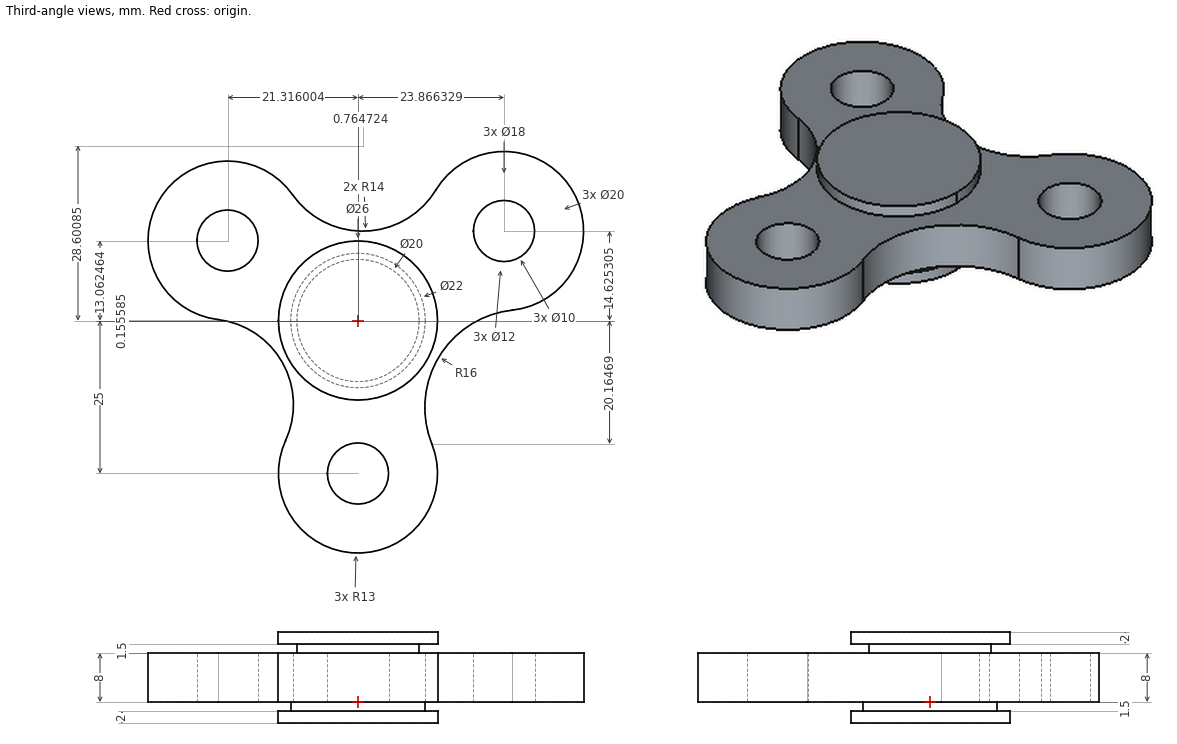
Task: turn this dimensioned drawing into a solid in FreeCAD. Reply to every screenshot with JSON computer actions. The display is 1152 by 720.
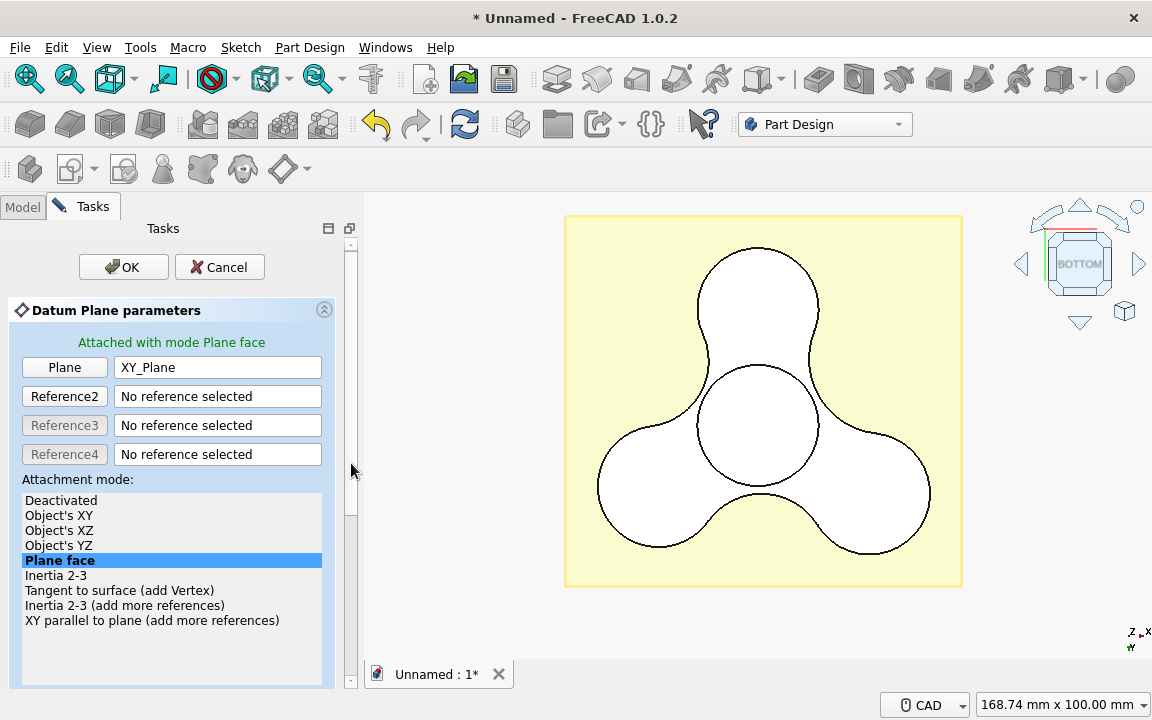
{"action": "left_click", "coordinate": [124, 267]}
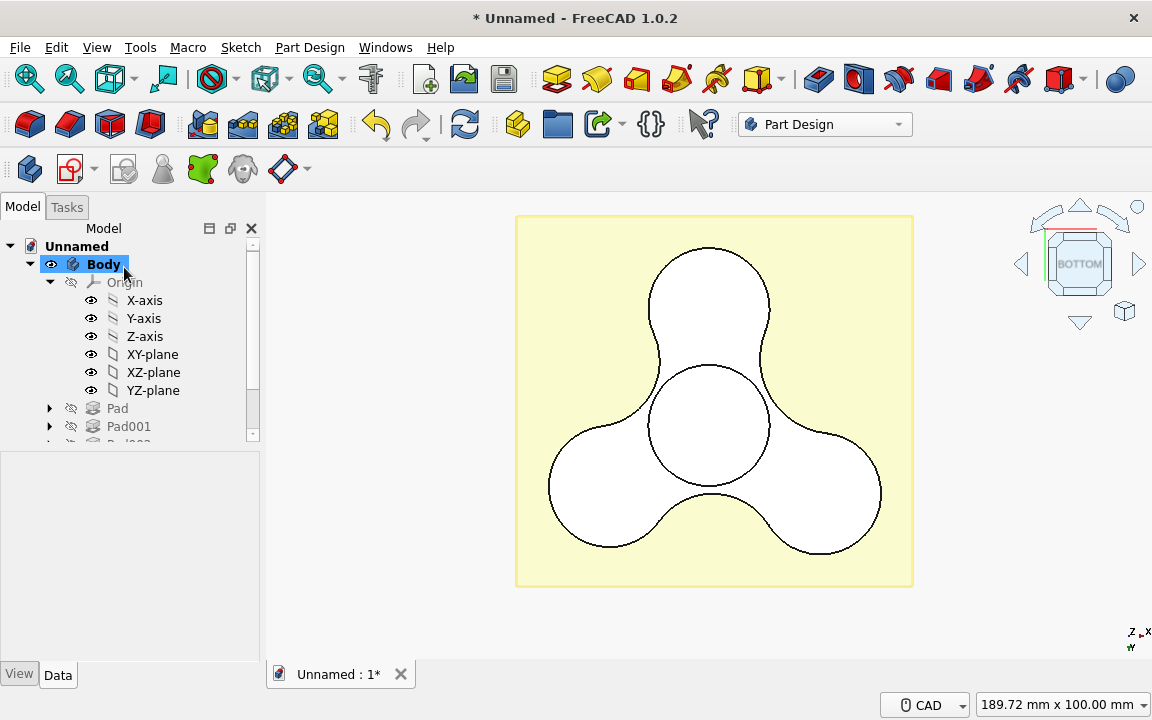
{"action": "scroll", "coordinate": [100, 332], "scroll_direction": "down", "scroll_amount": 3}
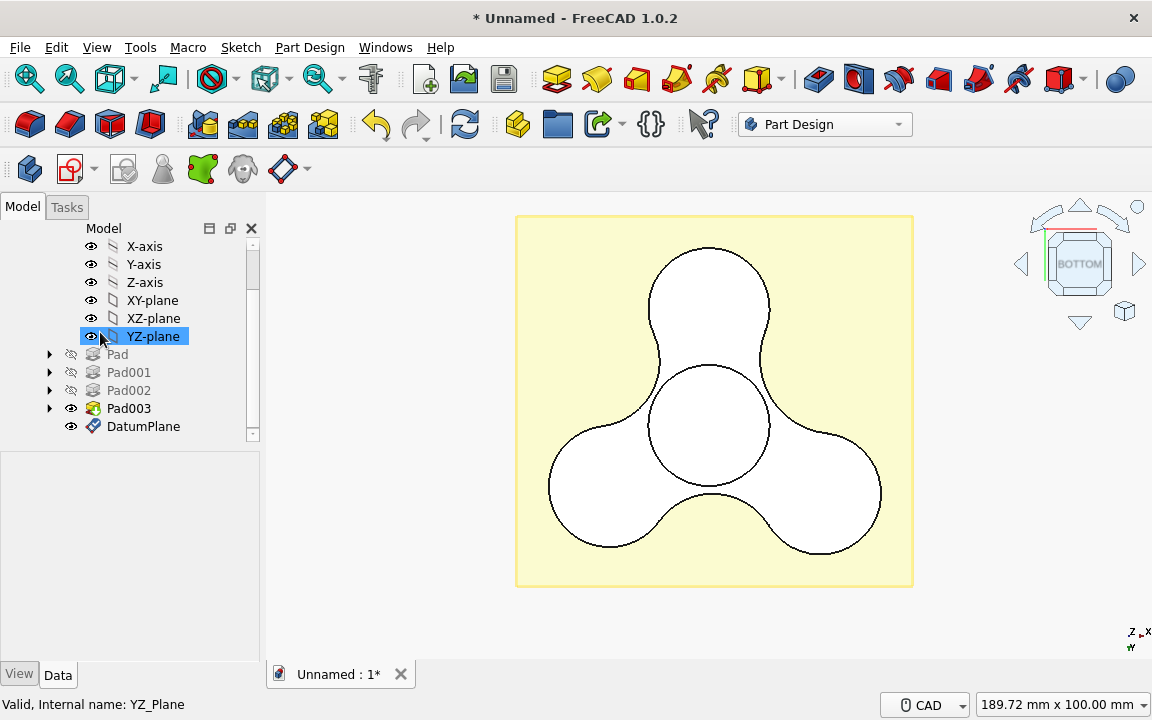
{"action": "left_click", "coordinate": [116, 426]}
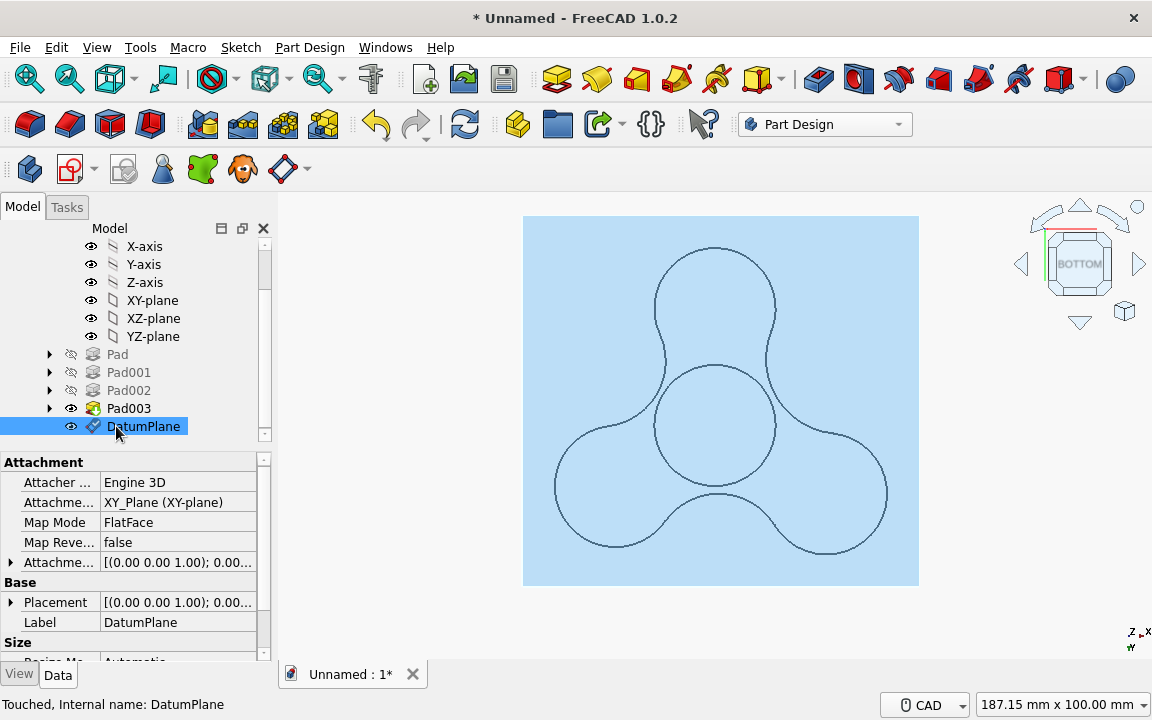
{"action": "left_click", "coordinate": [70, 170]}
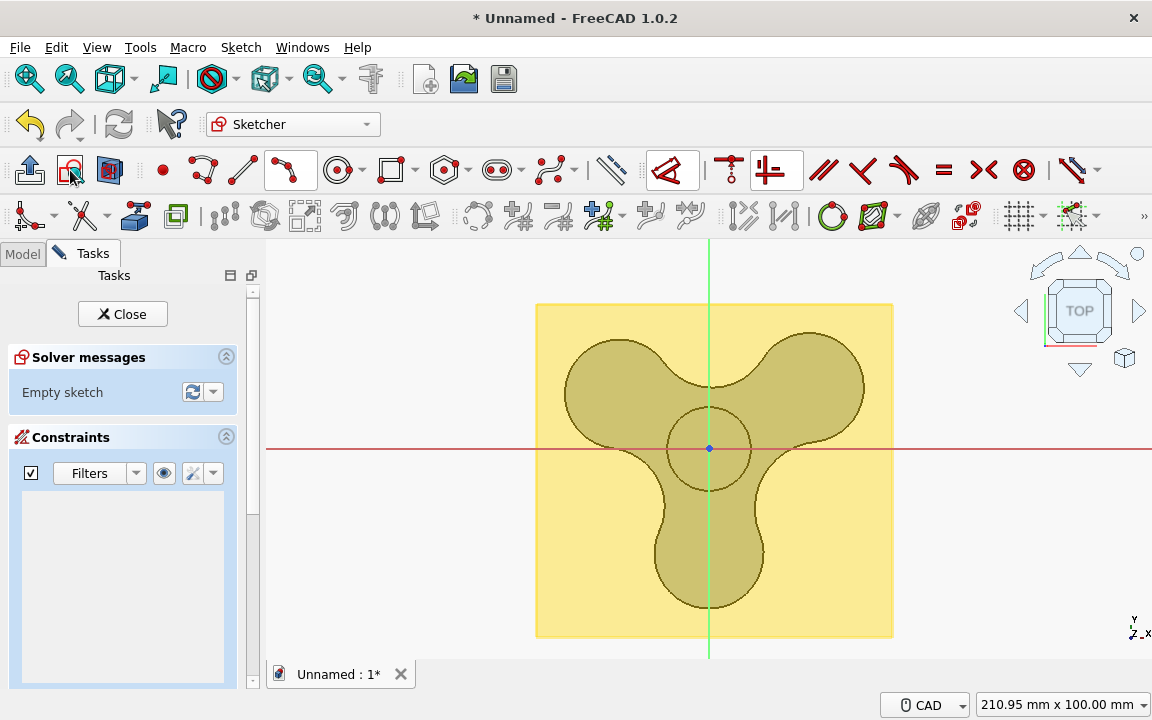
{"action": "scroll", "coordinate": [765, 449], "scroll_direction": "up", "scroll_amount": 4}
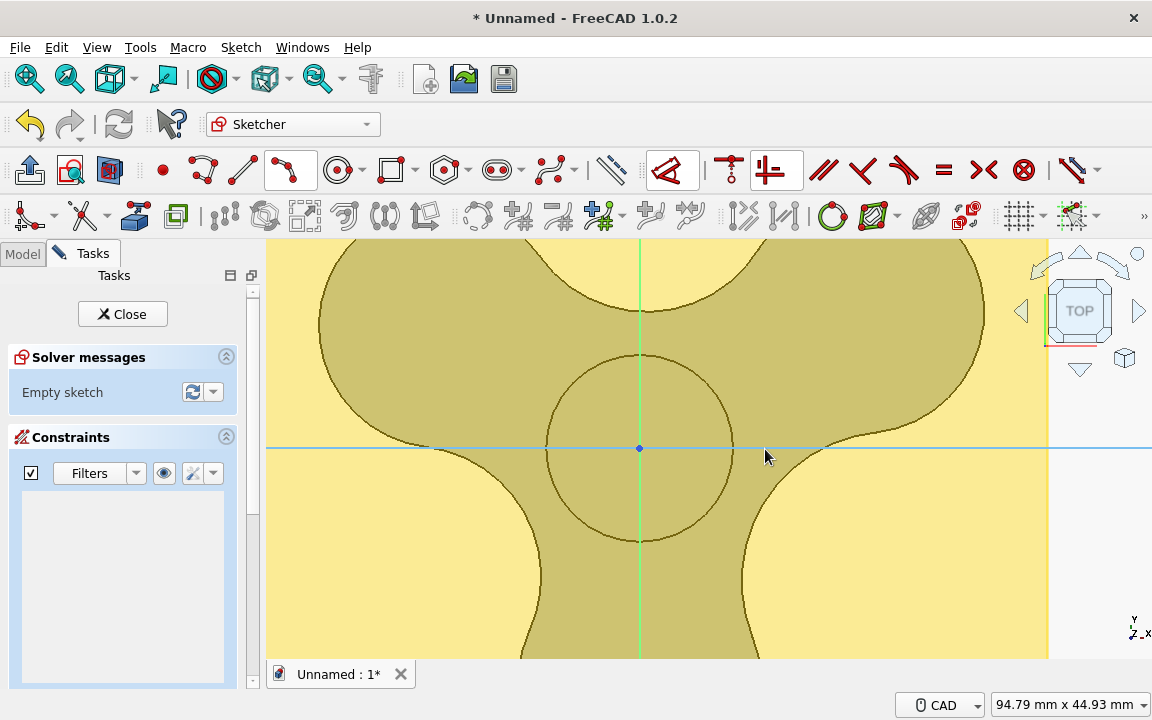
{"action": "left_click", "coordinate": [338, 170]}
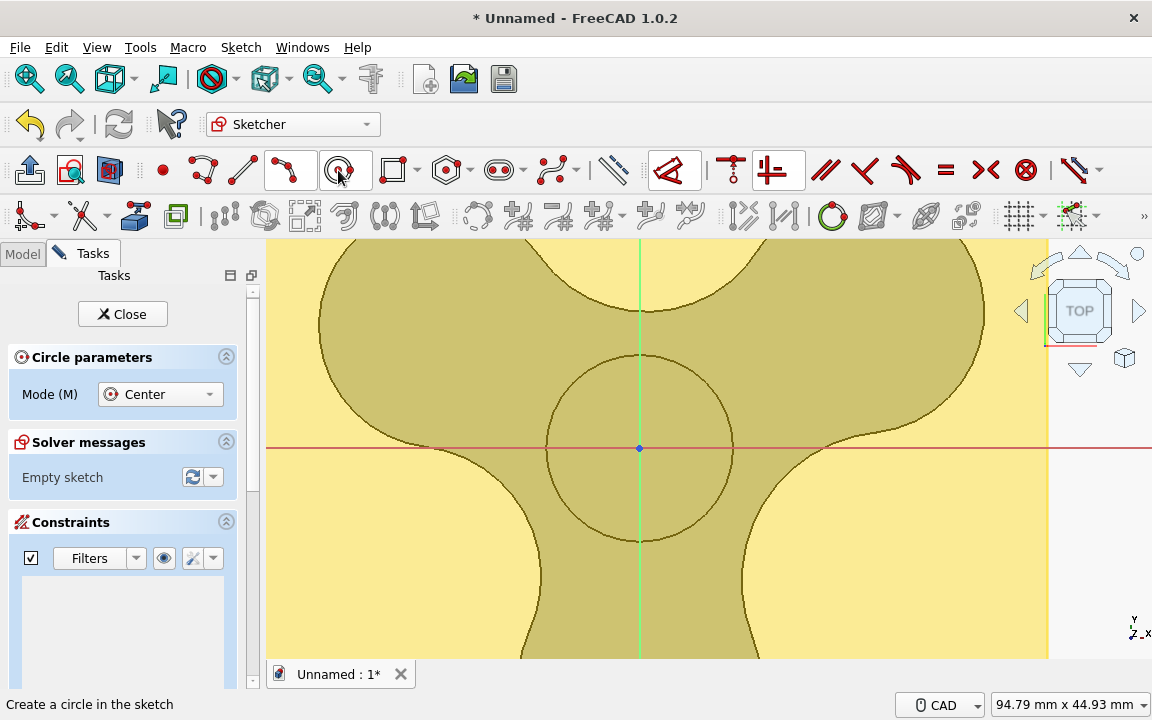
{"action": "left_click", "coordinate": [640, 448]}
{"action": "mouse_move", "coordinate": [726, 362]}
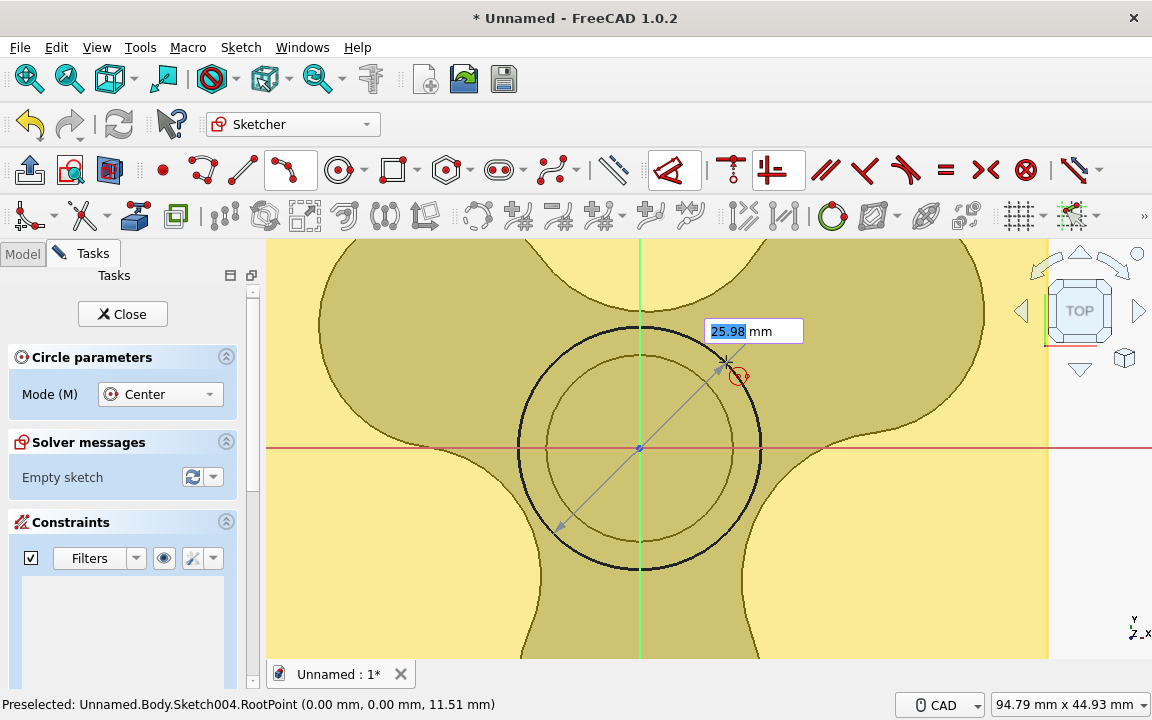
{"action": "type", "text": "26"}
{"action": "key", "text": "Return"}
{"action": "key", "text": "Escape"}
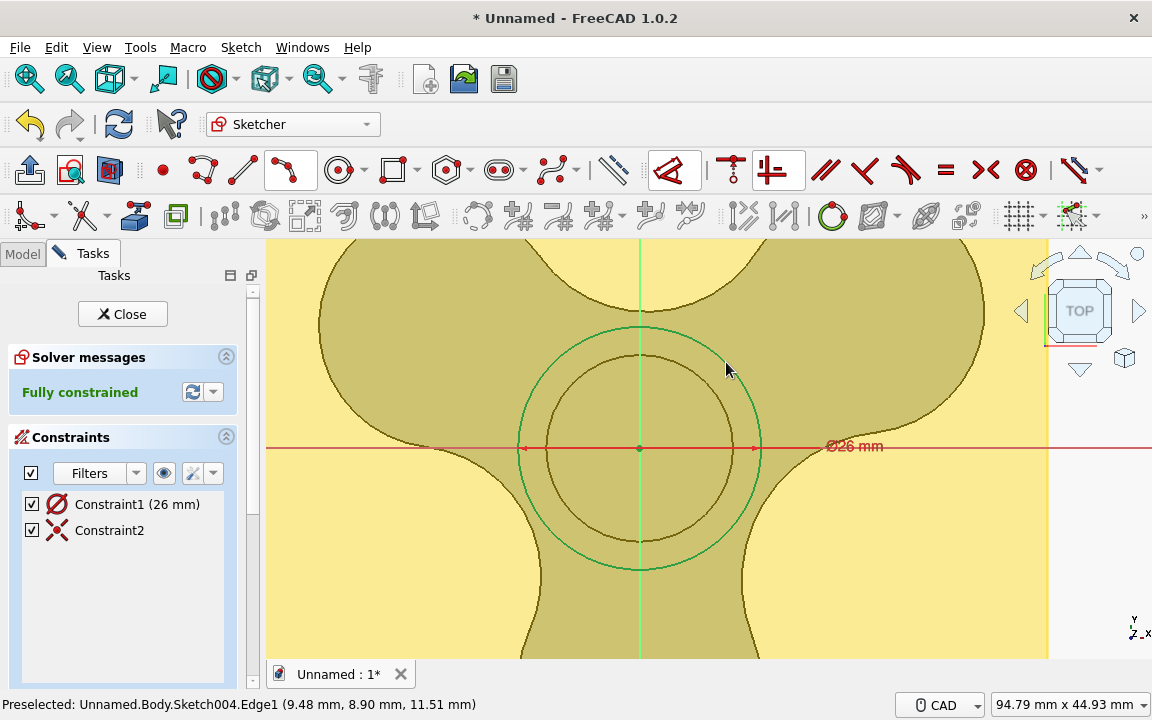
{"action": "left_click", "coordinate": [123, 314]}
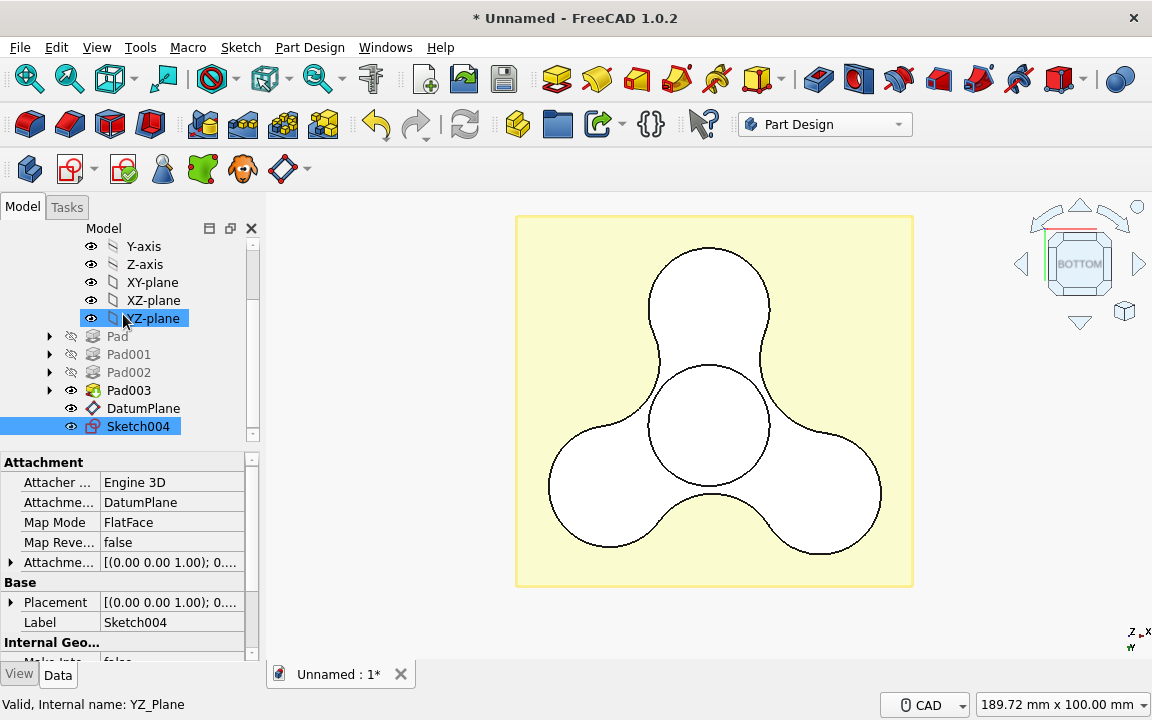
{"action": "left_click", "coordinate": [558, 80]}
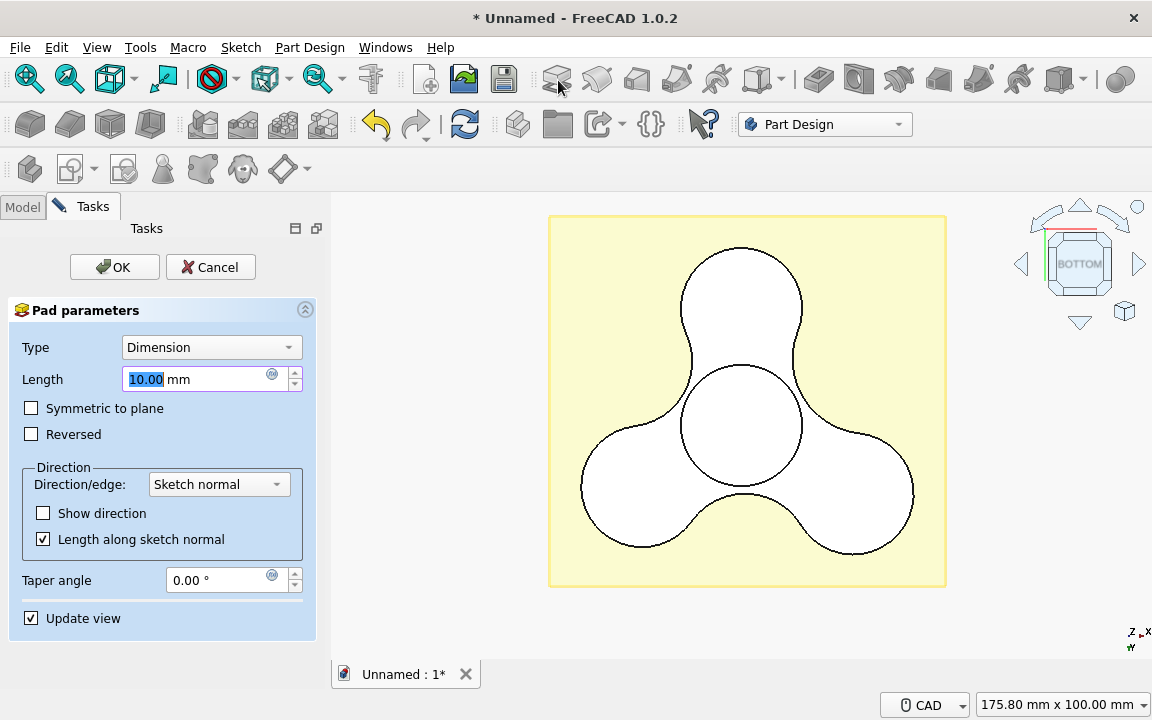
{"action": "type", "text": "2"}
{"action": "key", "text": "Tab"}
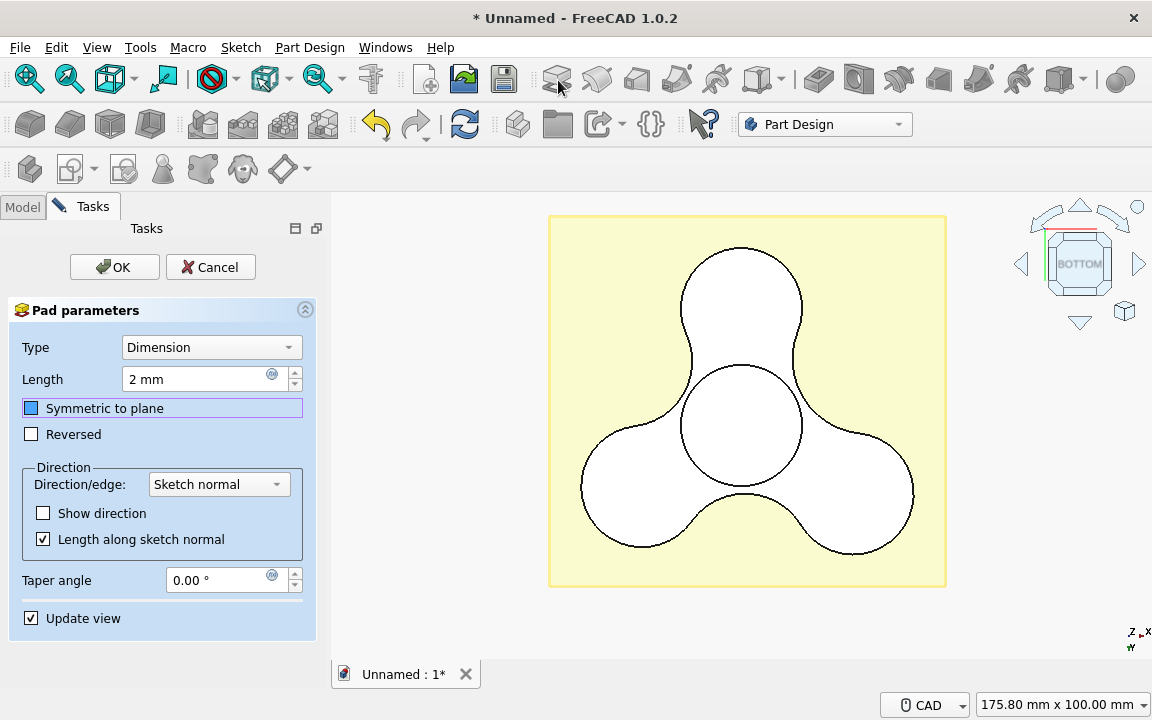
{"action": "left_click", "coordinate": [30, 434]}